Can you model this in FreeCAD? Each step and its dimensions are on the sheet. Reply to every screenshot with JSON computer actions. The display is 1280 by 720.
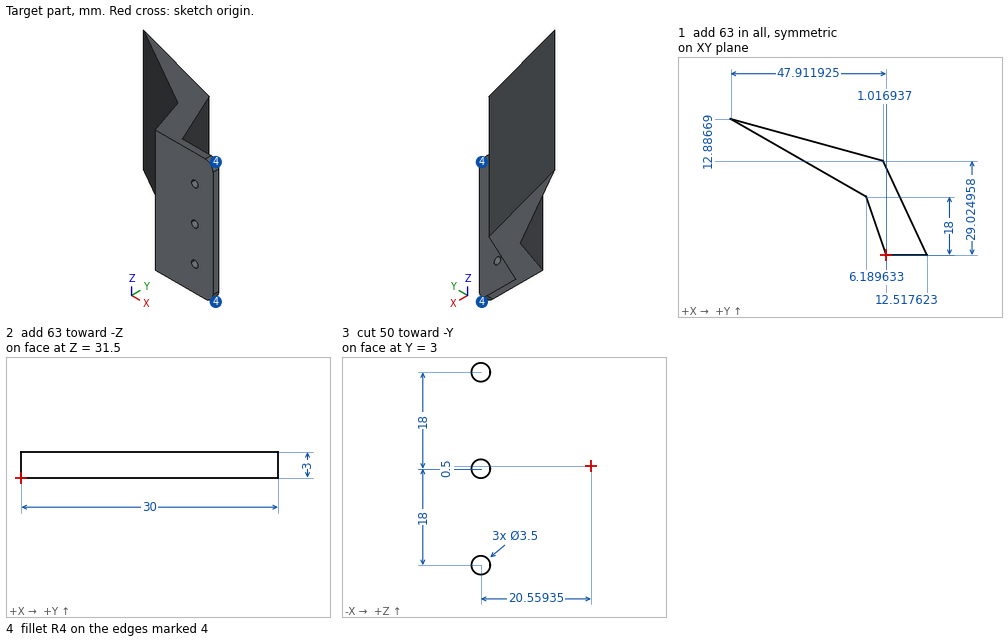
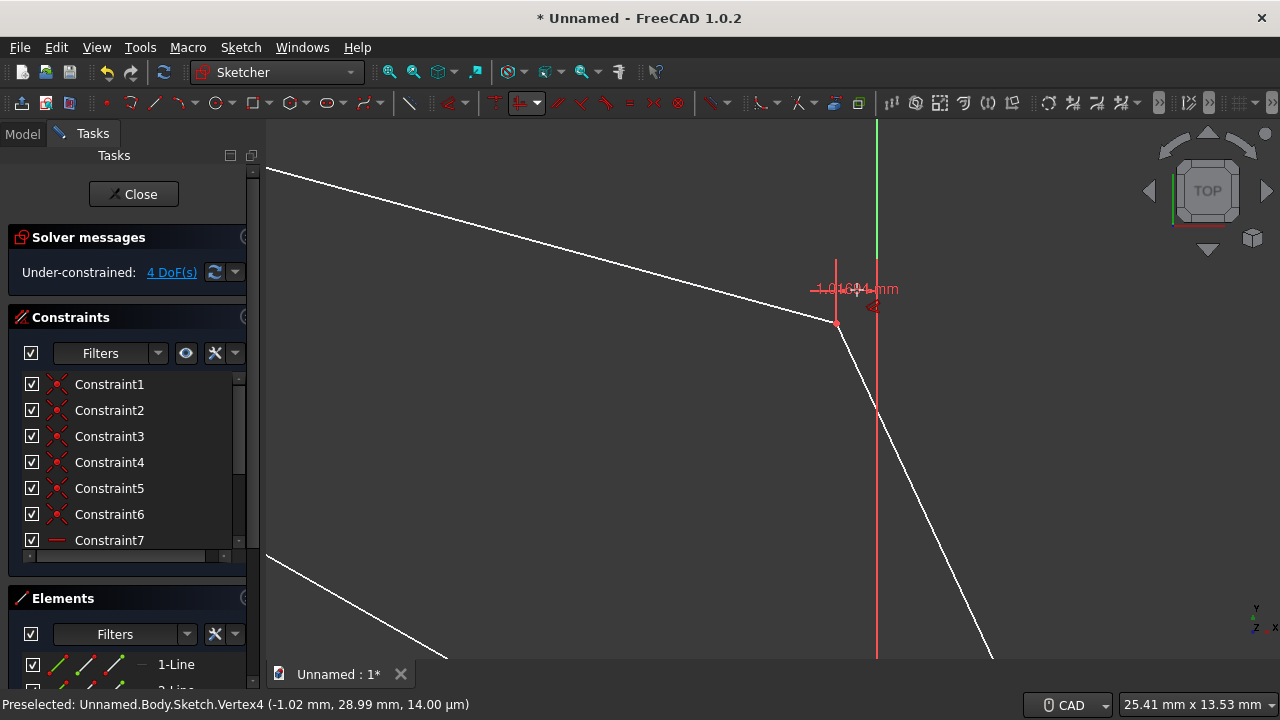
{"action": "scroll", "coordinate": [840, 324], "scroll_direction": "down", "scroll_amount": 8}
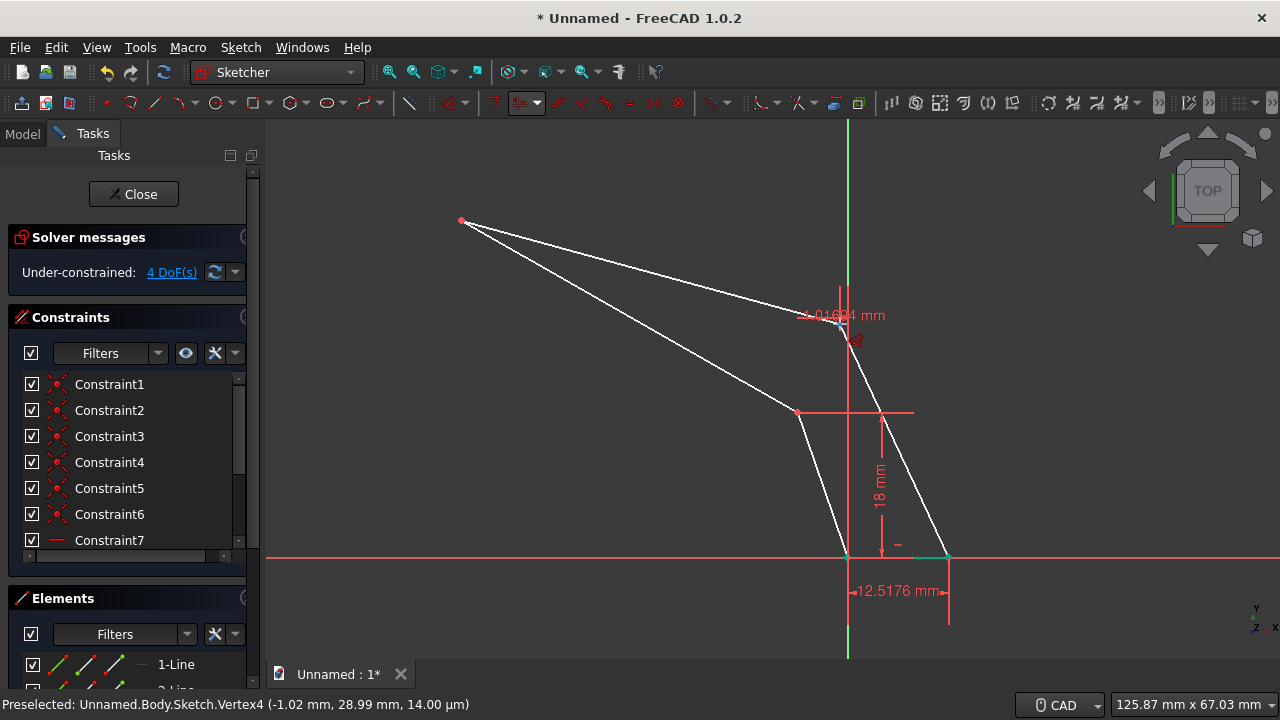
{"action": "left_click", "coordinate": [798, 413]}
{"action": "left_click", "coordinate": [823, 592]}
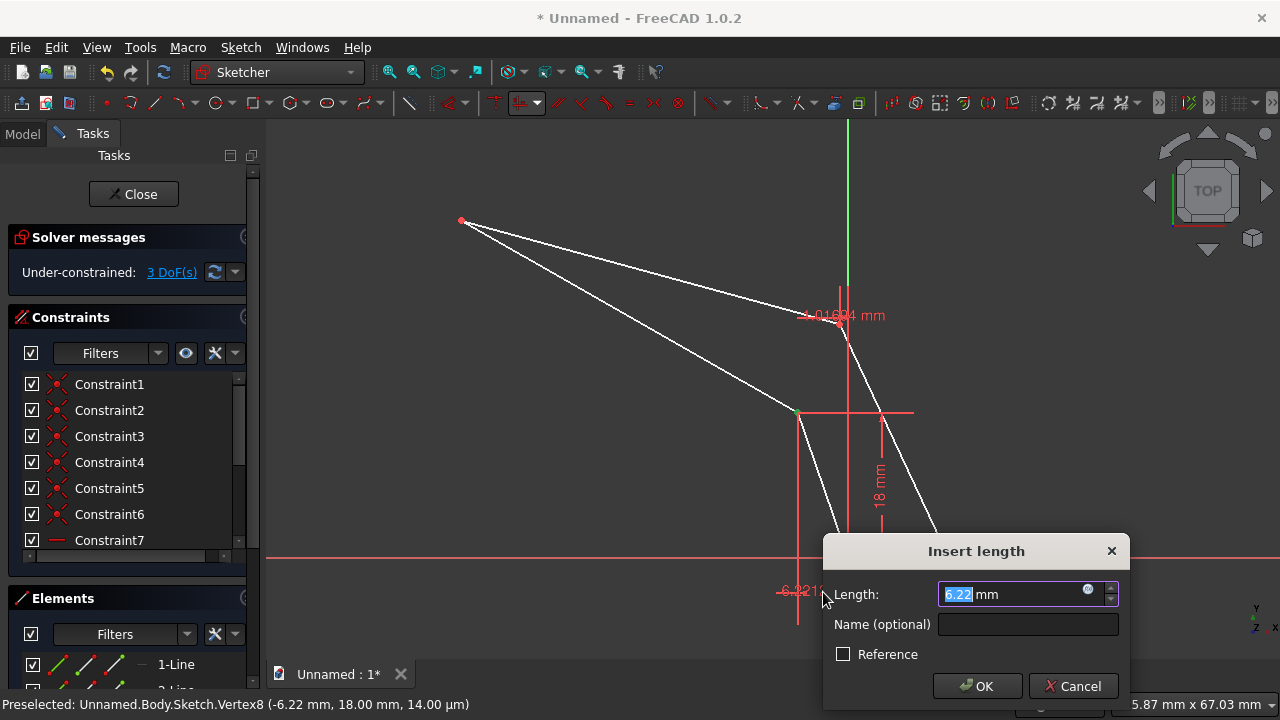
{"action": "type", "text": "6.189633"}
{"action": "key", "text": "Return"}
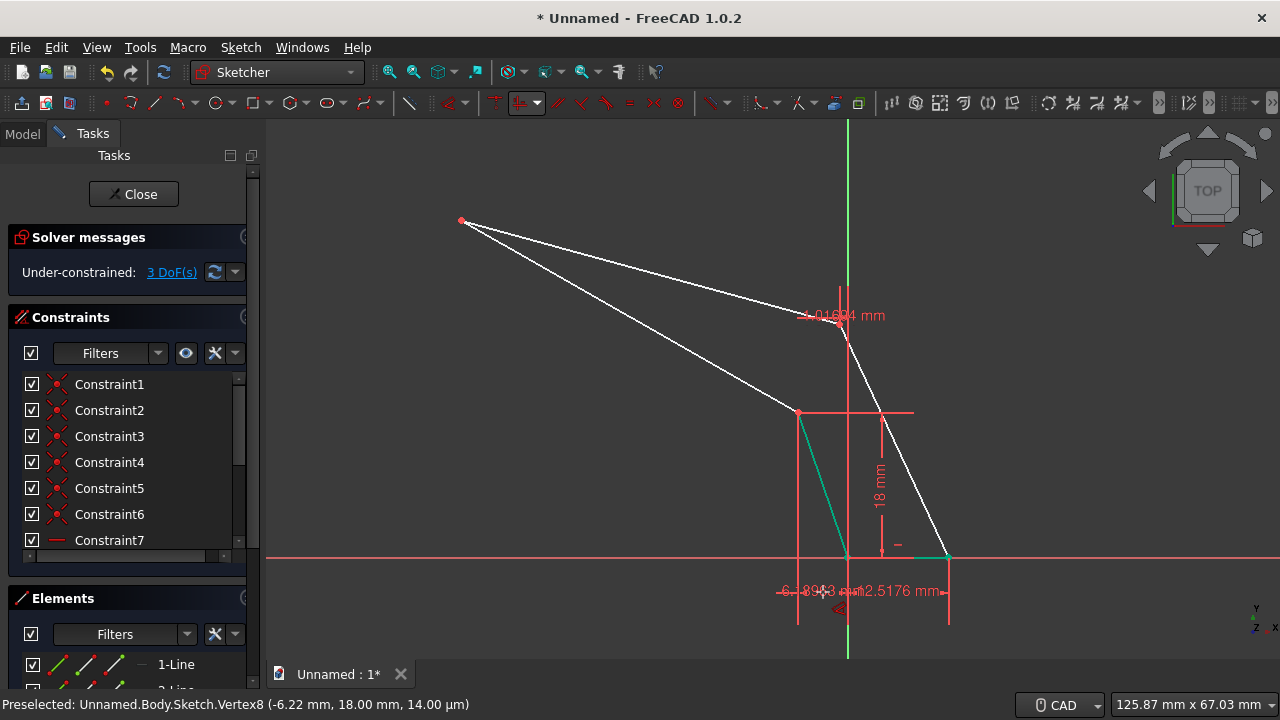
{"action": "left_click", "coordinate": [726, 293]}
{"action": "left_click", "coordinate": [428, 273]}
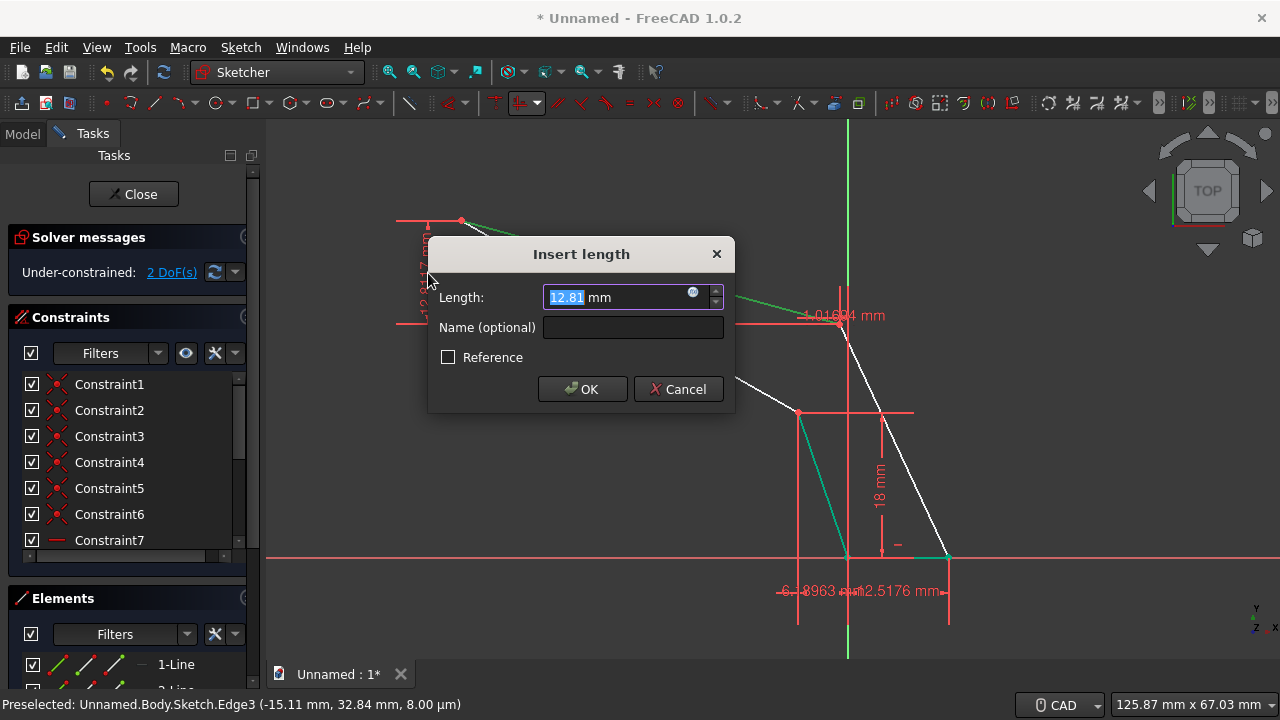
{"action": "type", "text": "12.88669"}
{"action": "key", "text": "Return"}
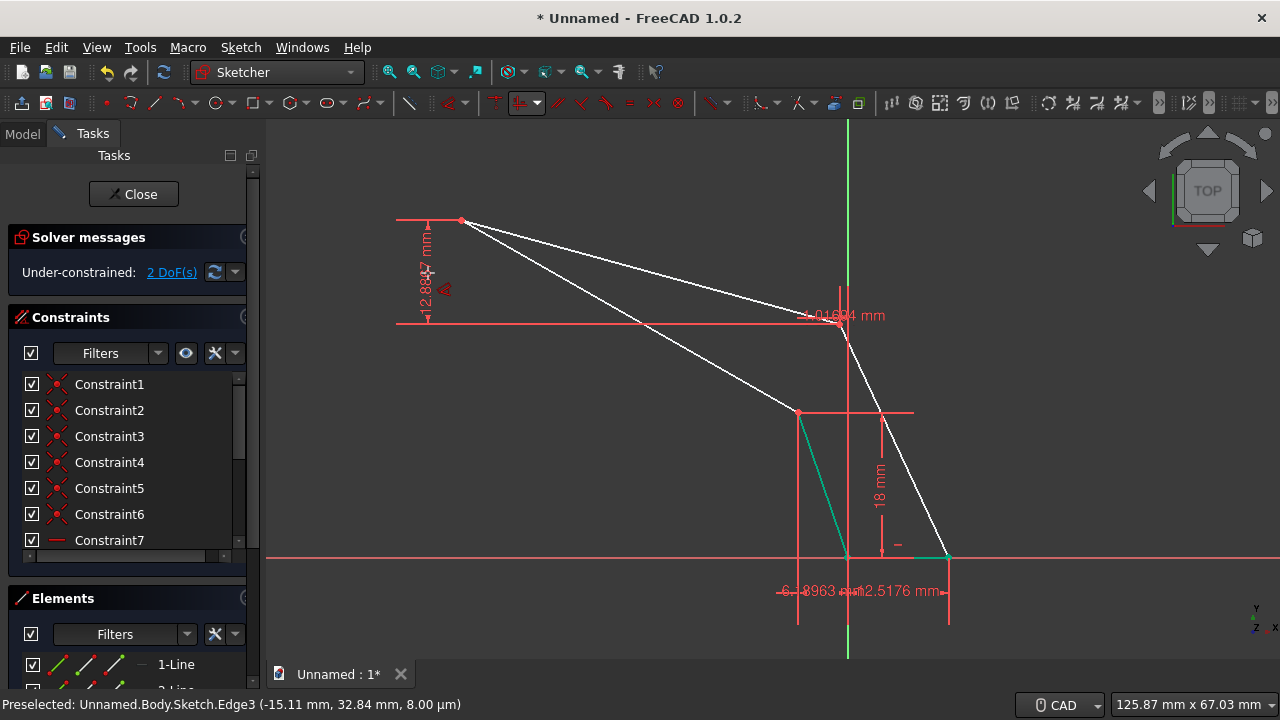
{"action": "left_click", "coordinate": [840, 324]}
{"action": "left_click", "coordinate": [882, 359]}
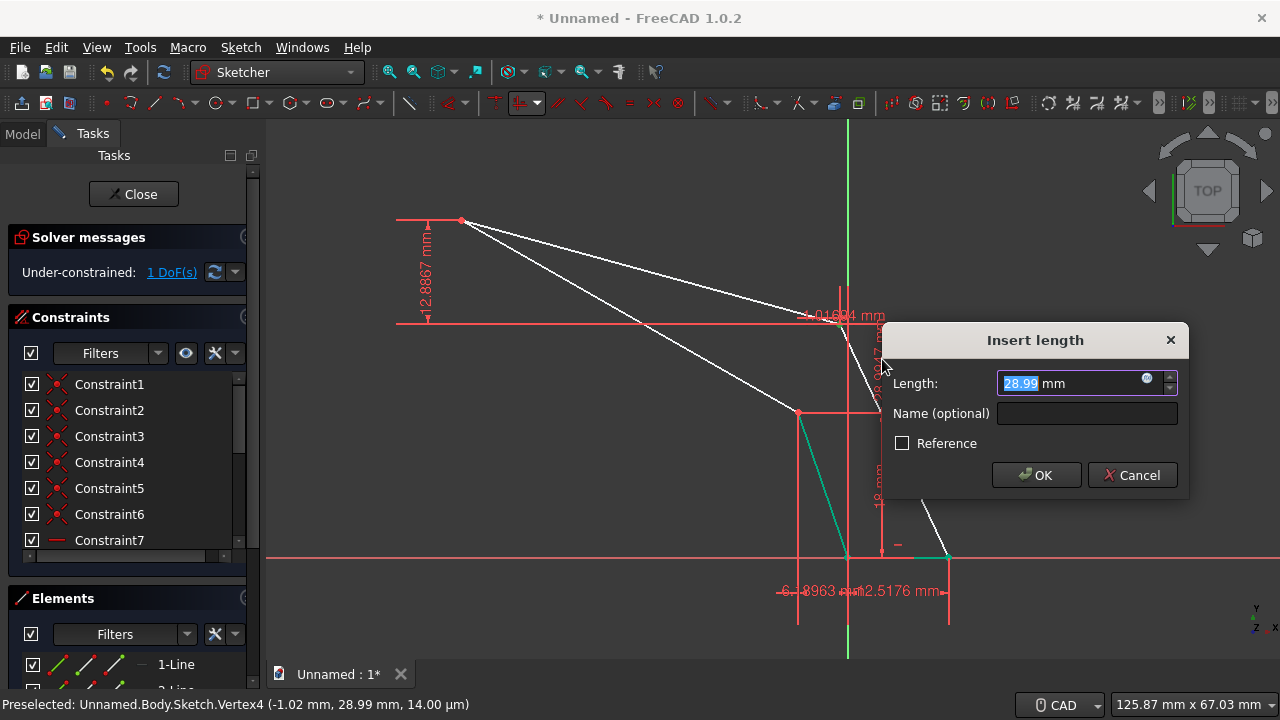
{"action": "type", "text": "29.024958"}
{"action": "key", "text": "Return"}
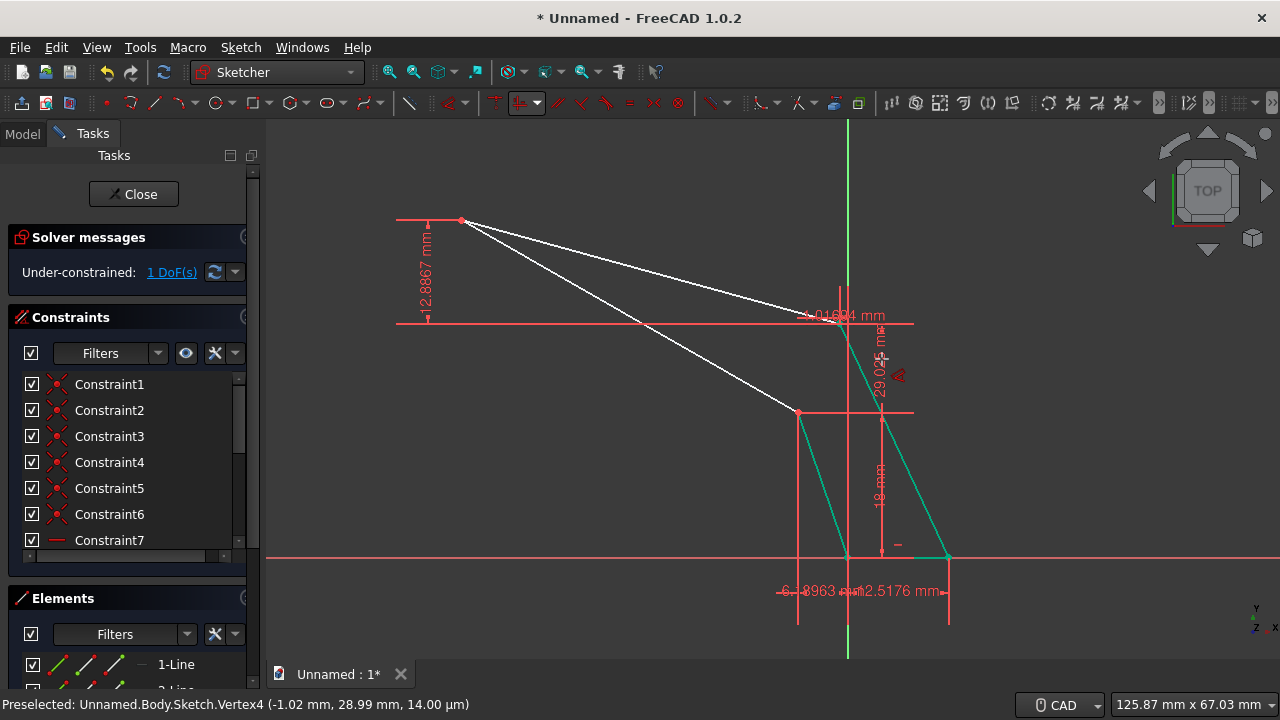
{"action": "left_click", "coordinate": [462, 220]}
{"action": "left_click", "coordinate": [655, 592]}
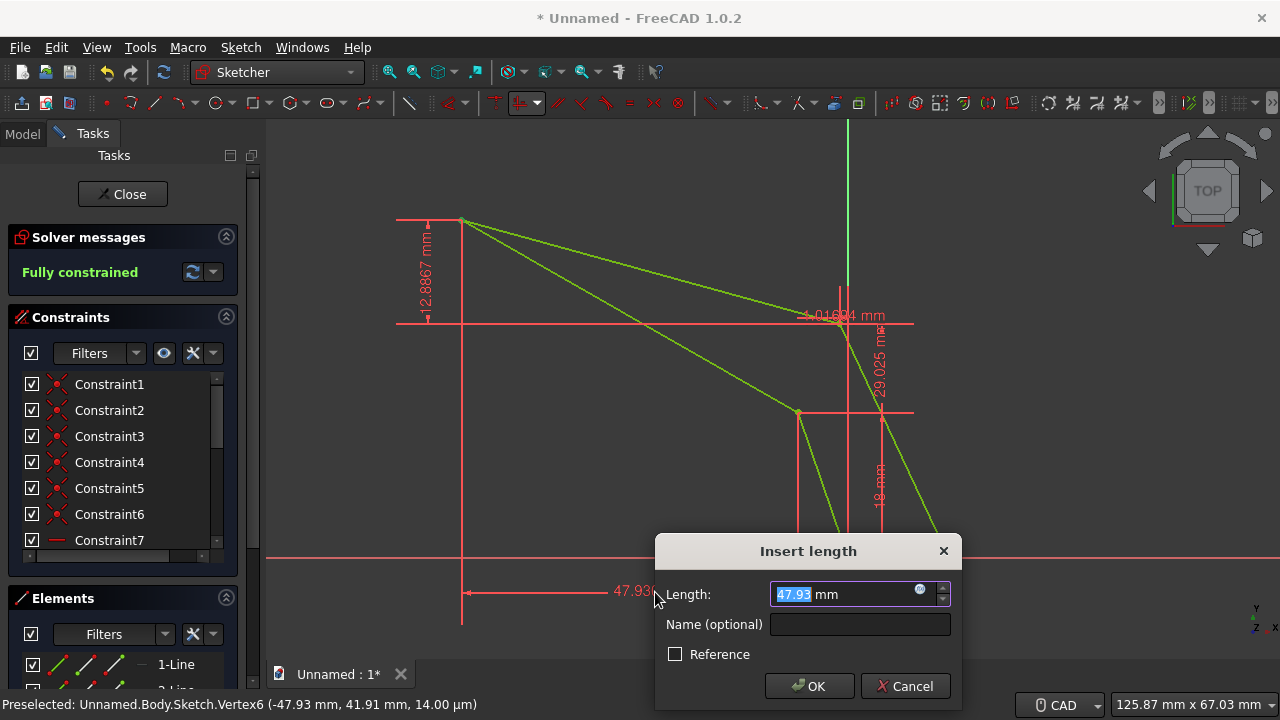
{"action": "type", "text": "47.911925"}
{"action": "key", "text": "Return"}
{"action": "key", "text": "Escape"}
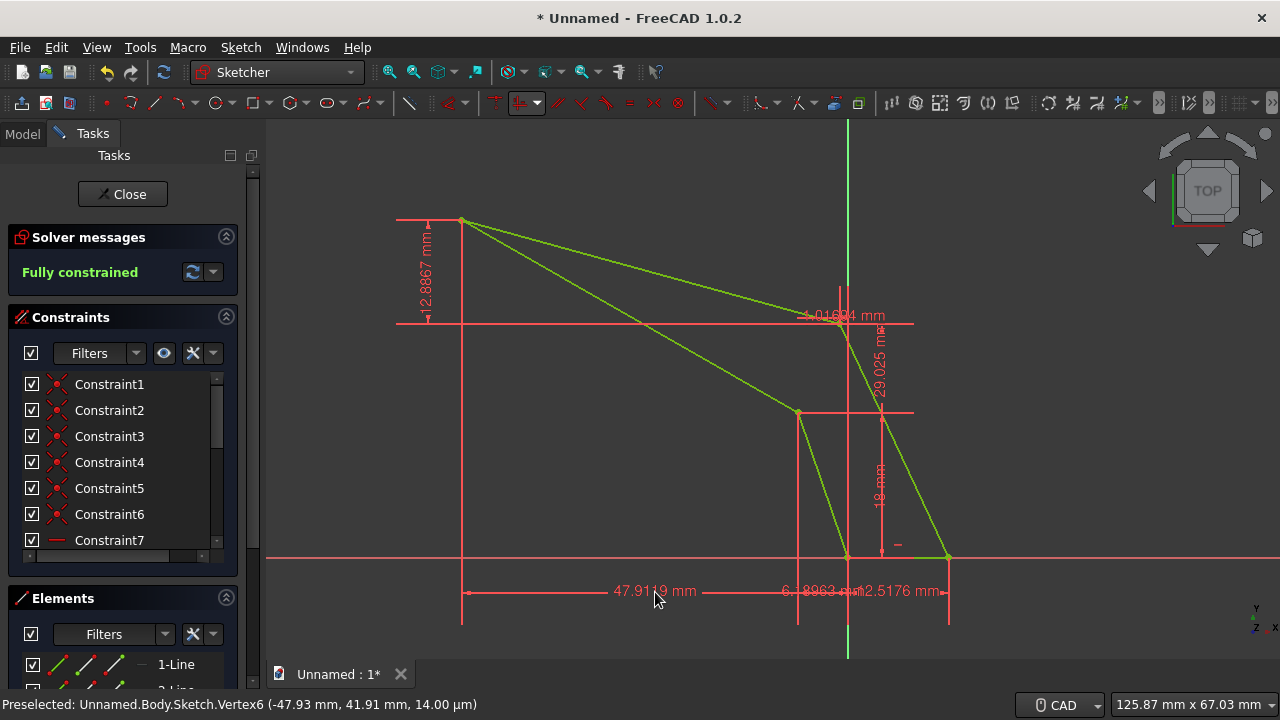
{"action": "left_click", "coordinate": [123, 194]}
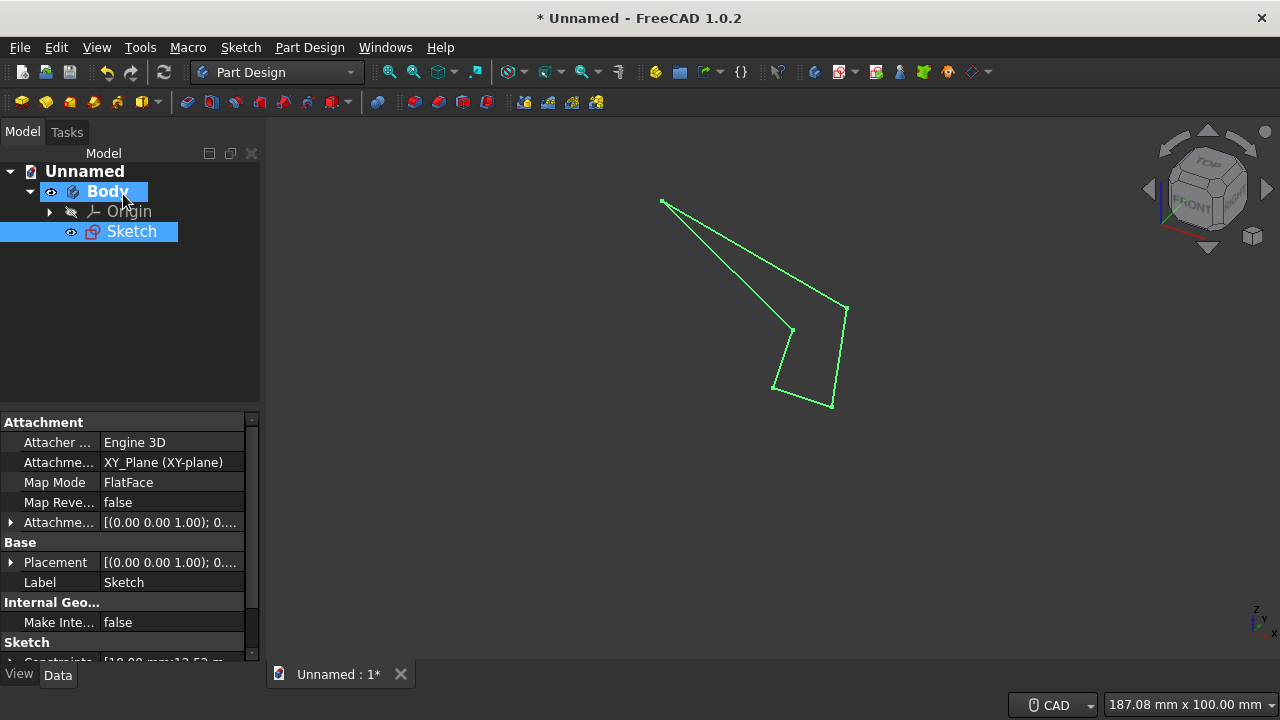
{"action": "left_click", "coordinate": [22, 102]}